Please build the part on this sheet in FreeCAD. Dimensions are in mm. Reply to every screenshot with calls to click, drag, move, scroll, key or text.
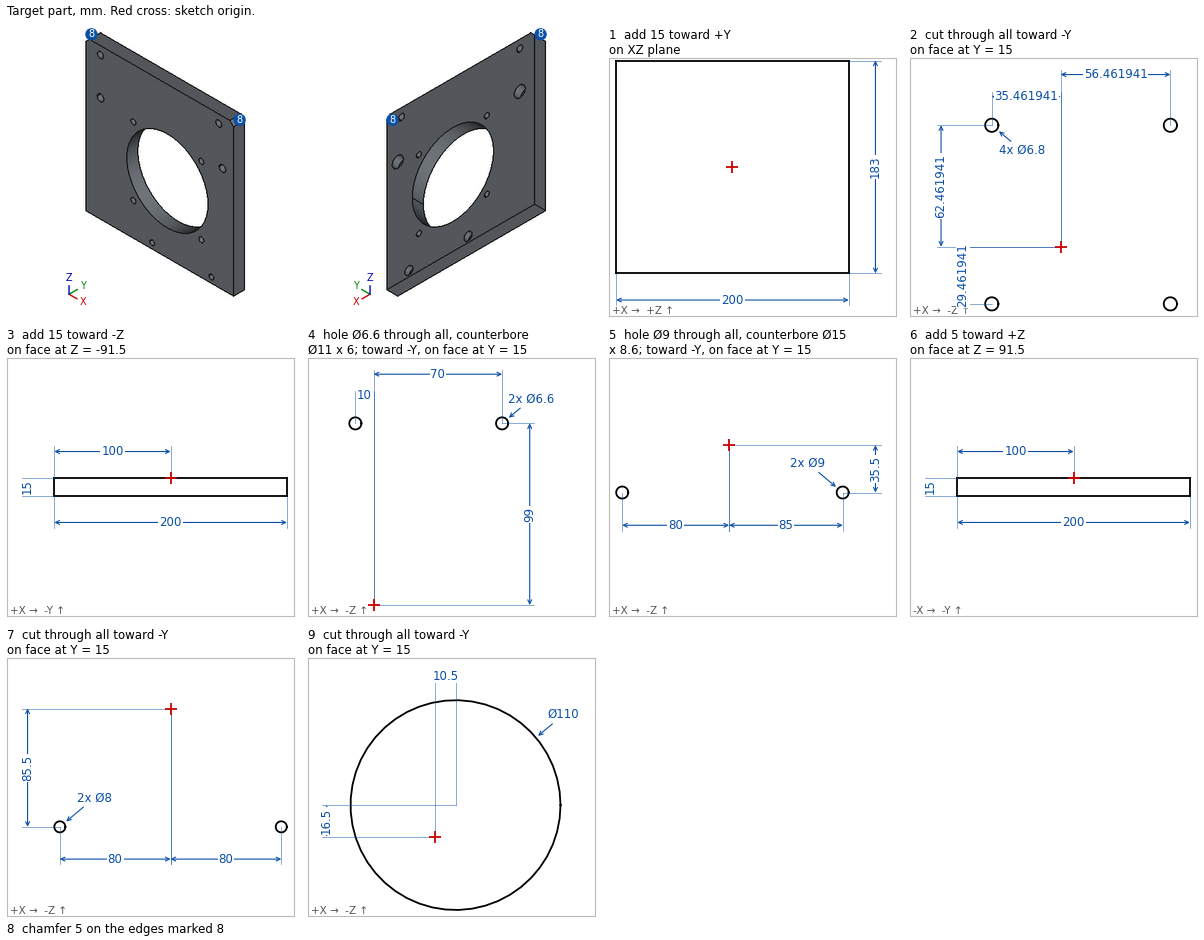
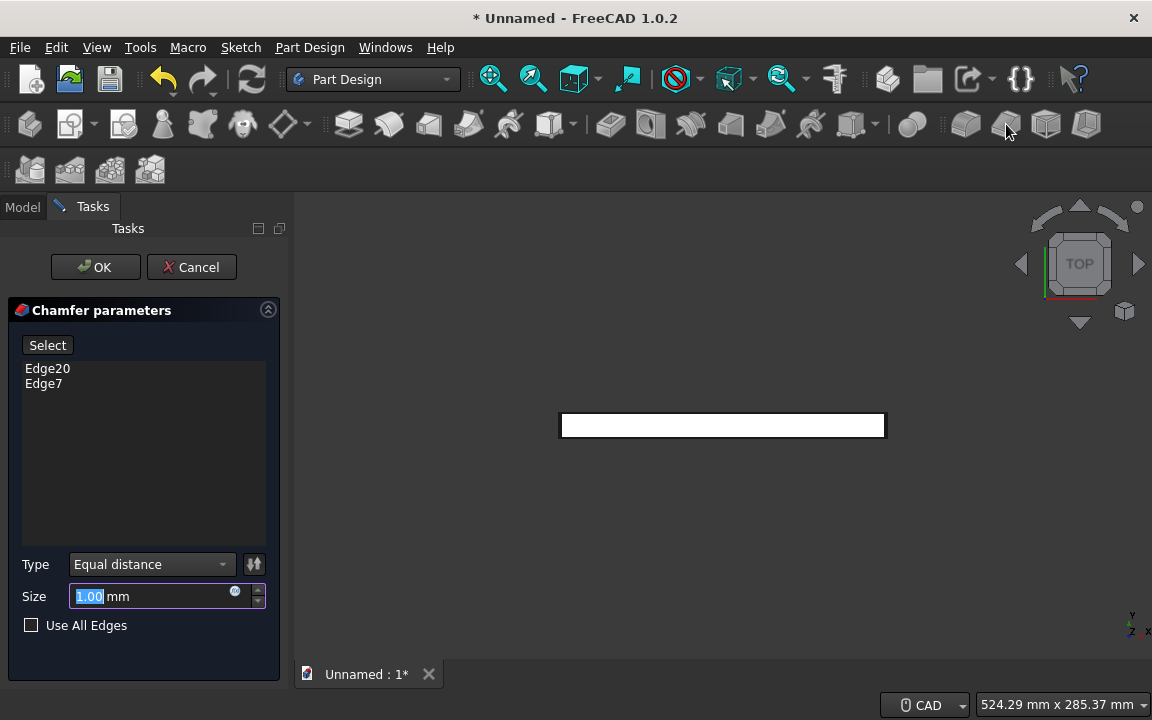
text(5)
key(Tab)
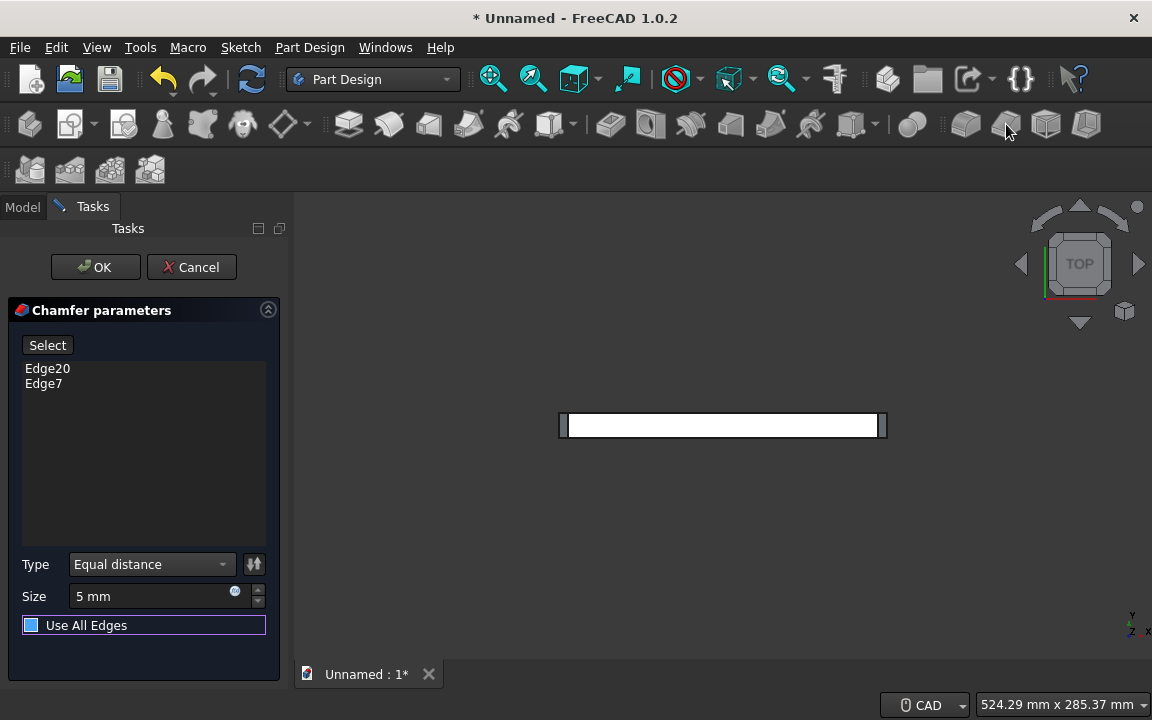
click(96, 267)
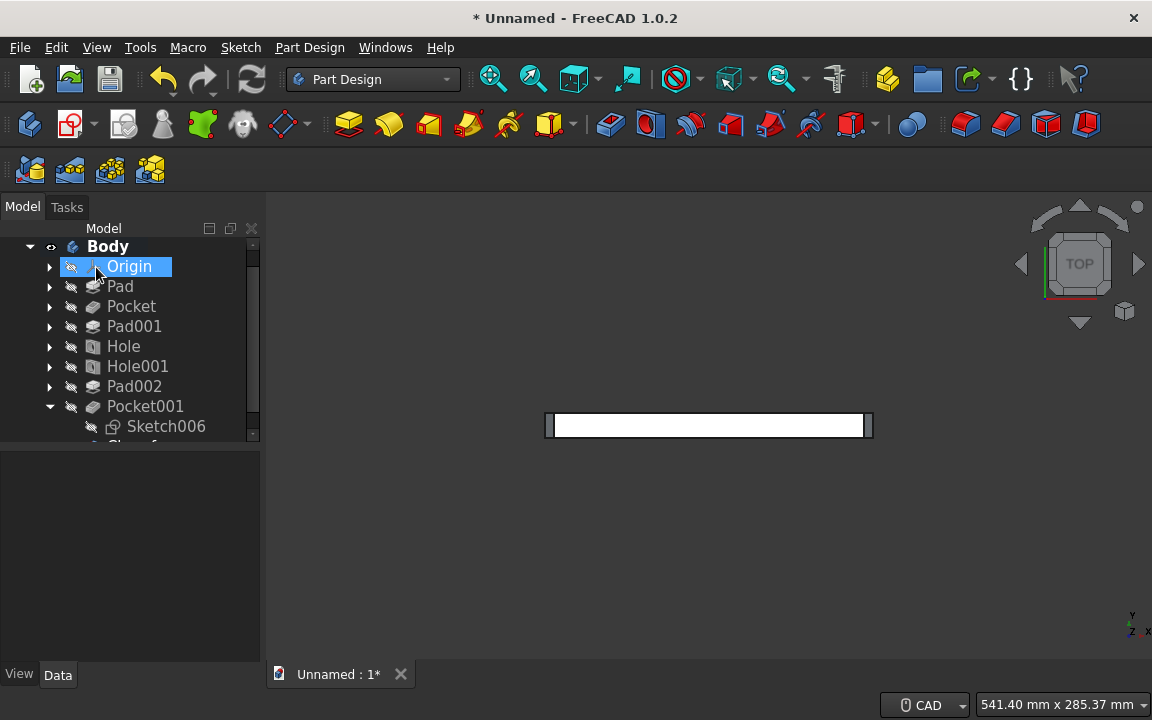
click(494, 80)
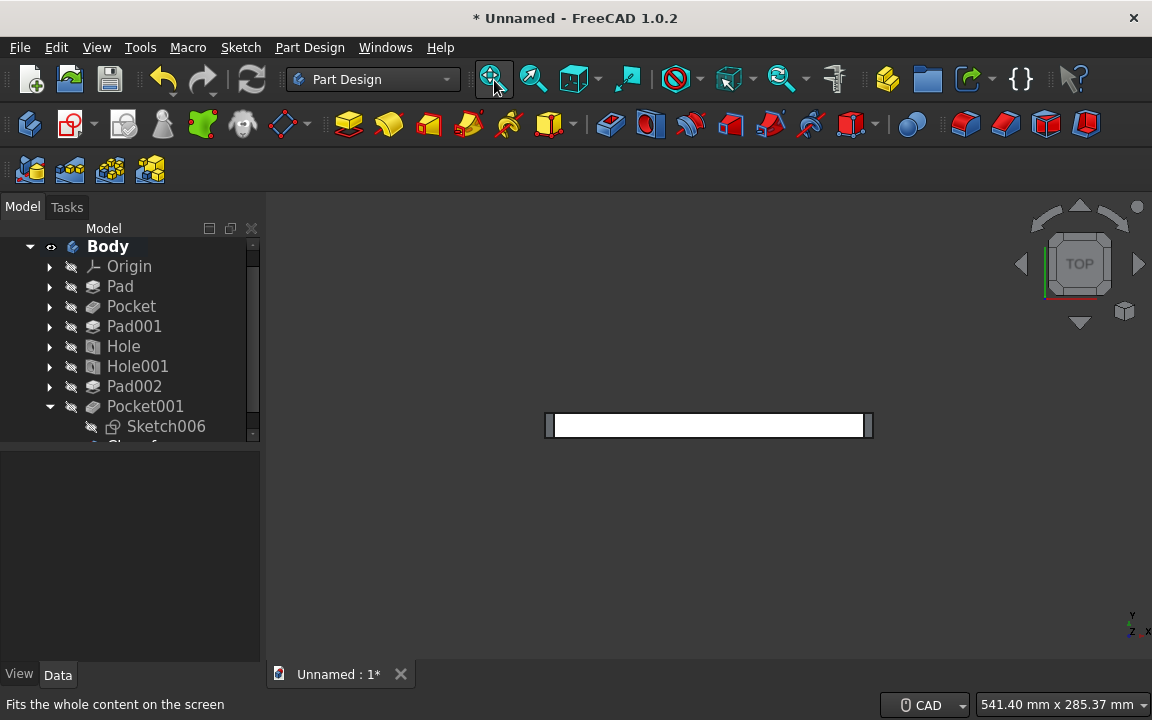
key(4)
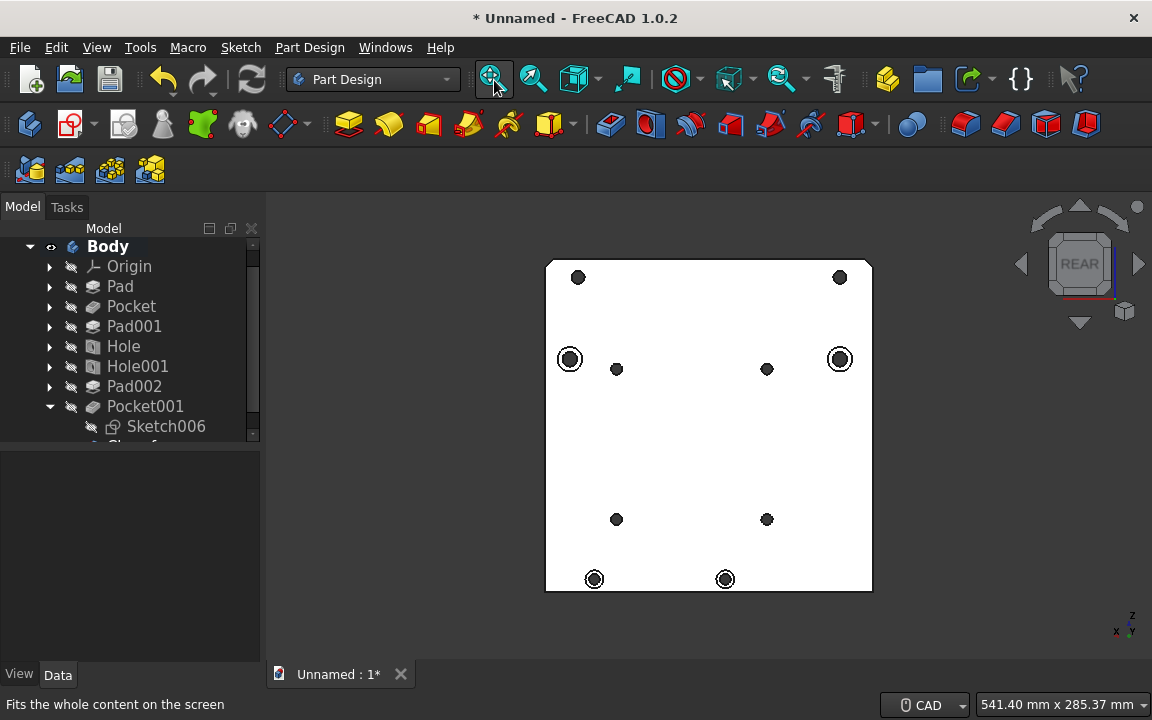
click(709, 425)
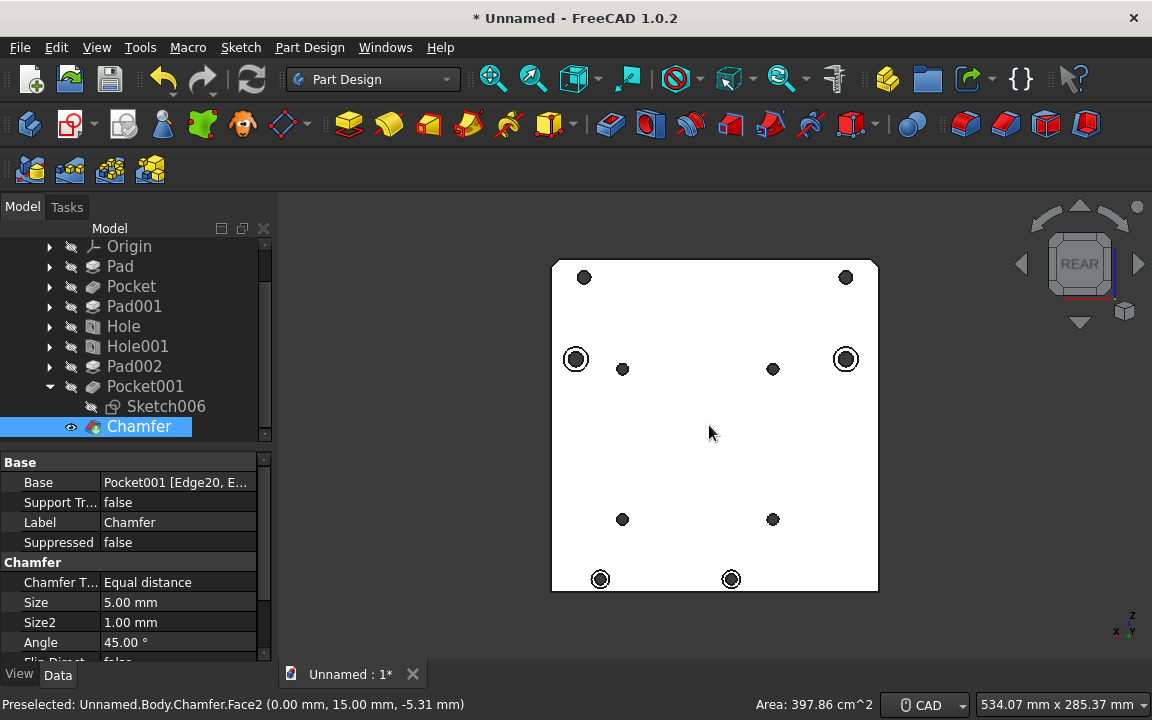
click(70, 124)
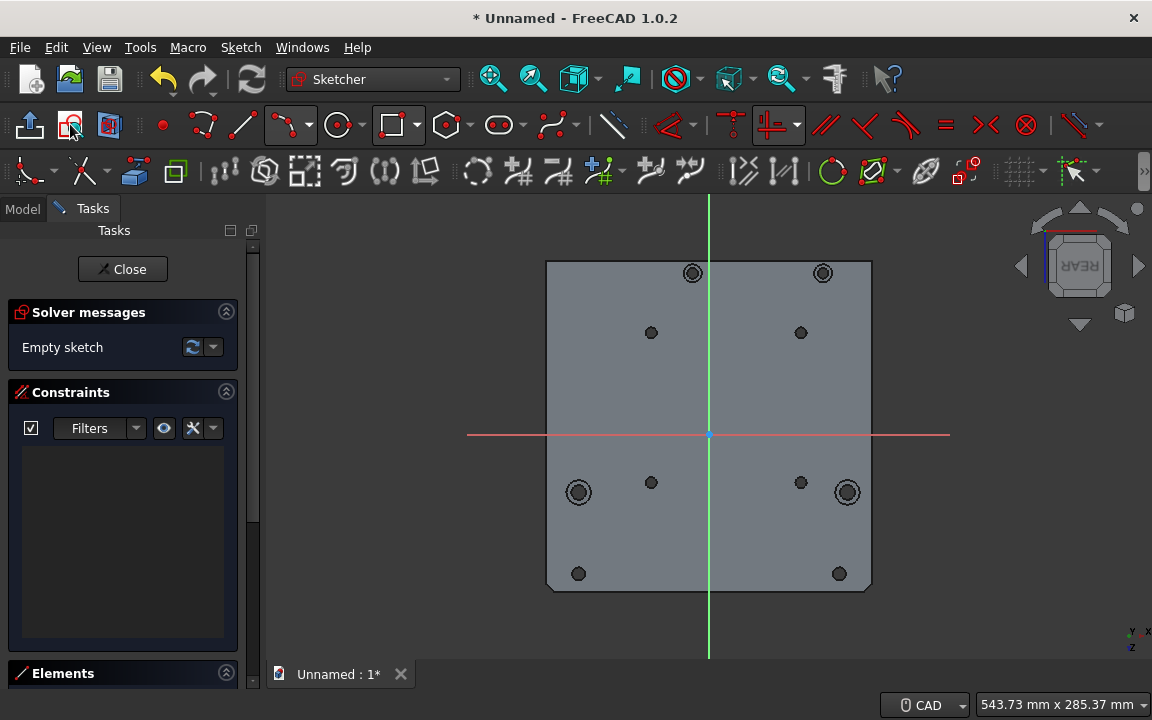
scroll(900, 370, up, 2)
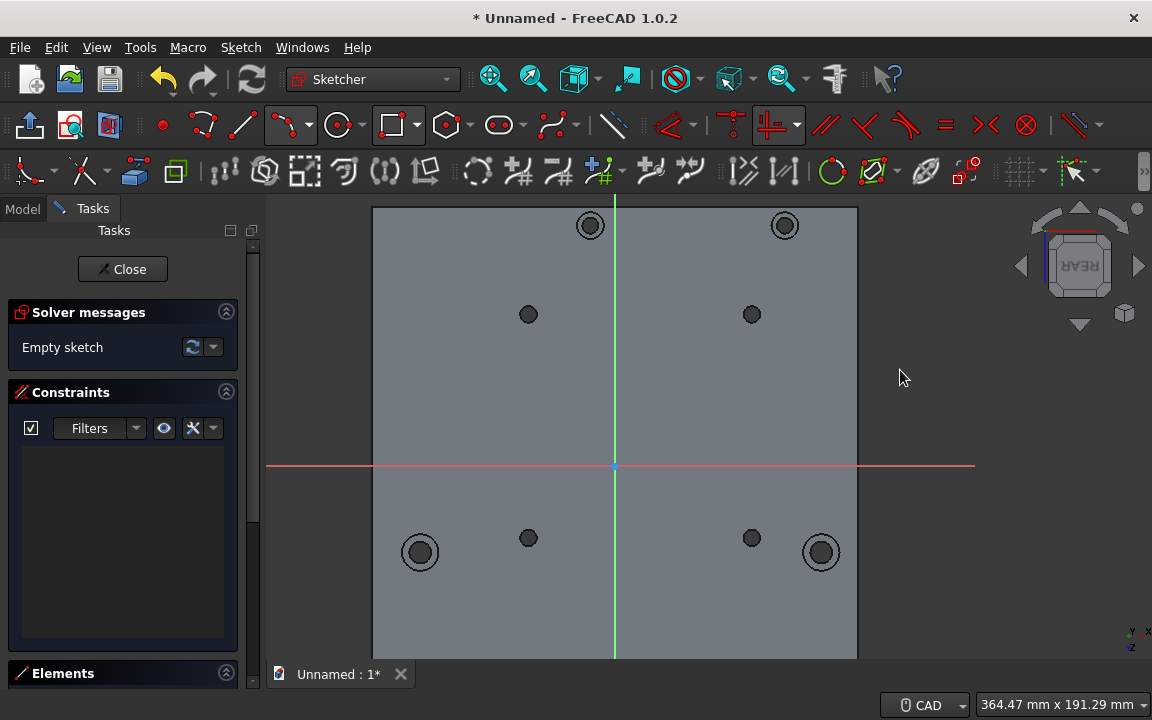
click(338, 126)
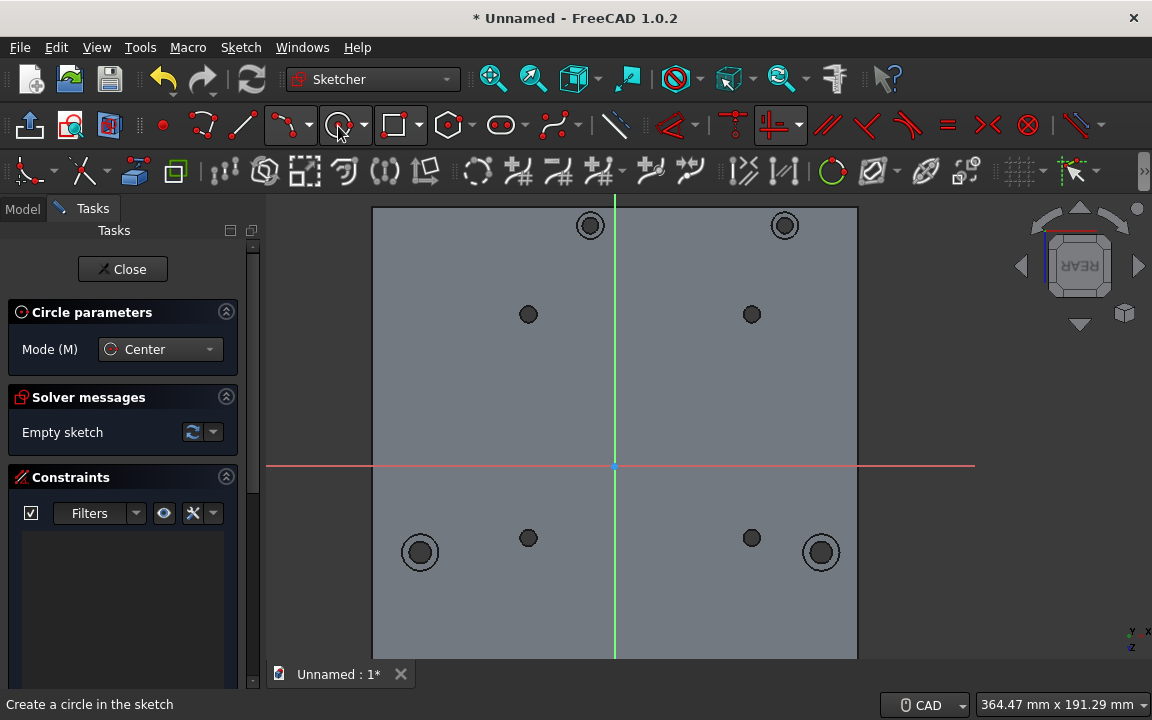
click(640, 426)
click(735, 332)
key(Escape)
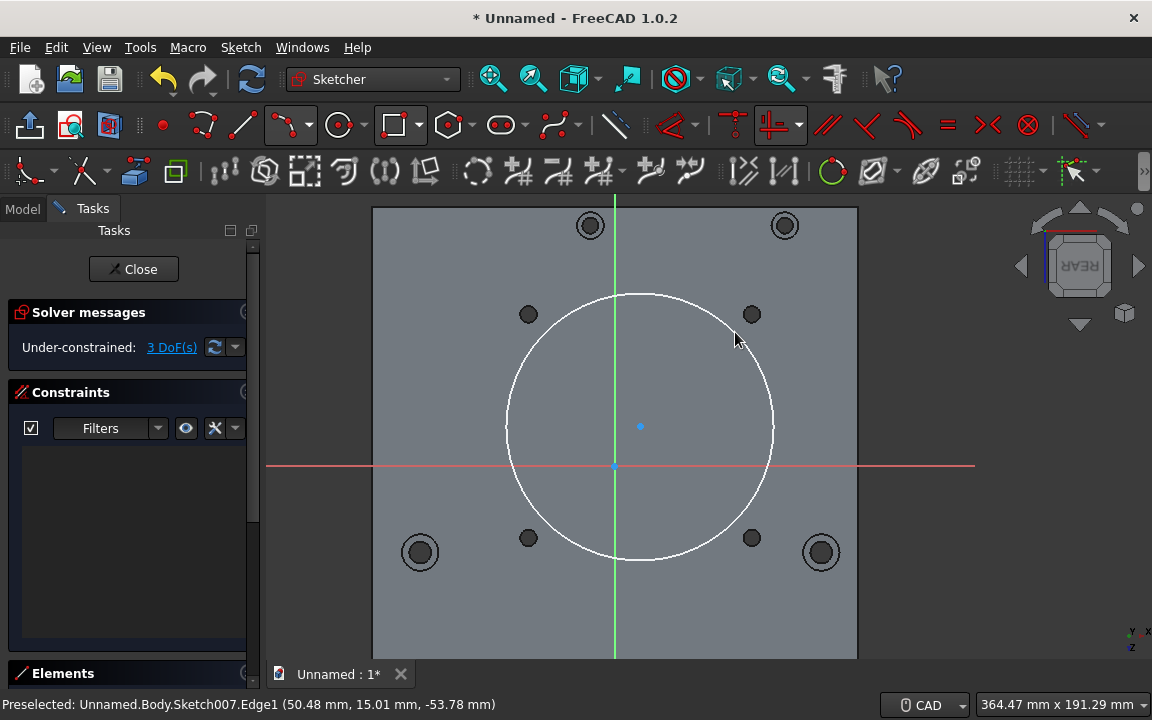
click(670, 126)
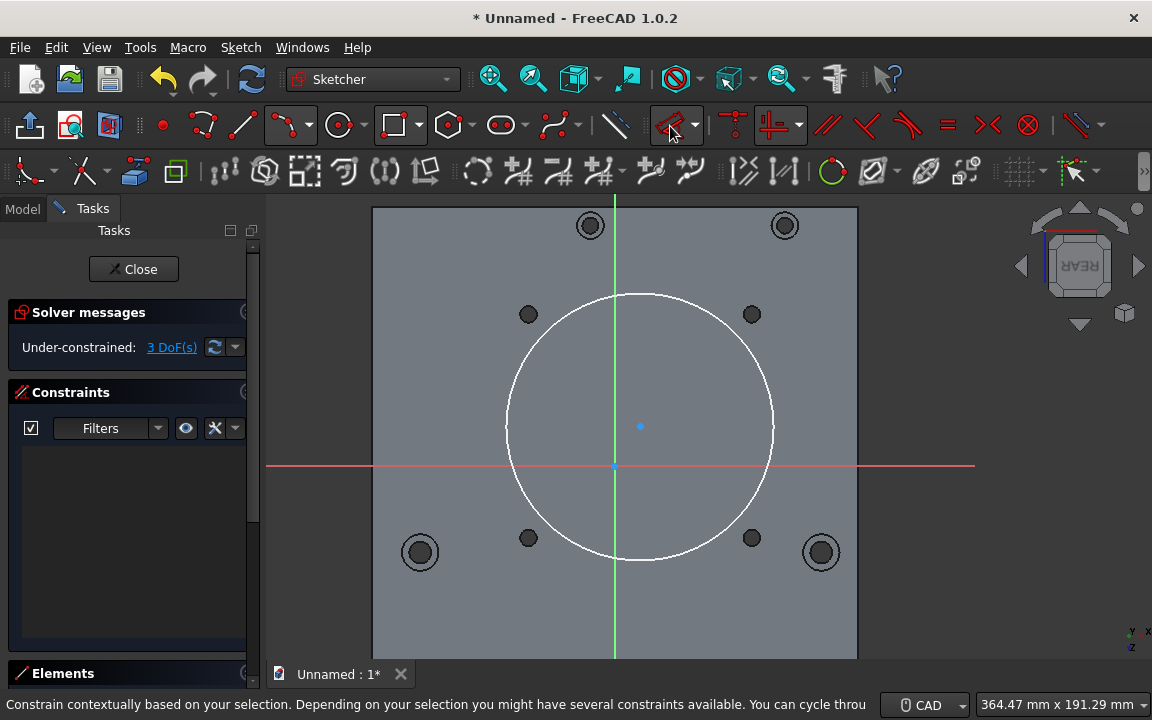
click(734, 332)
click(757, 309)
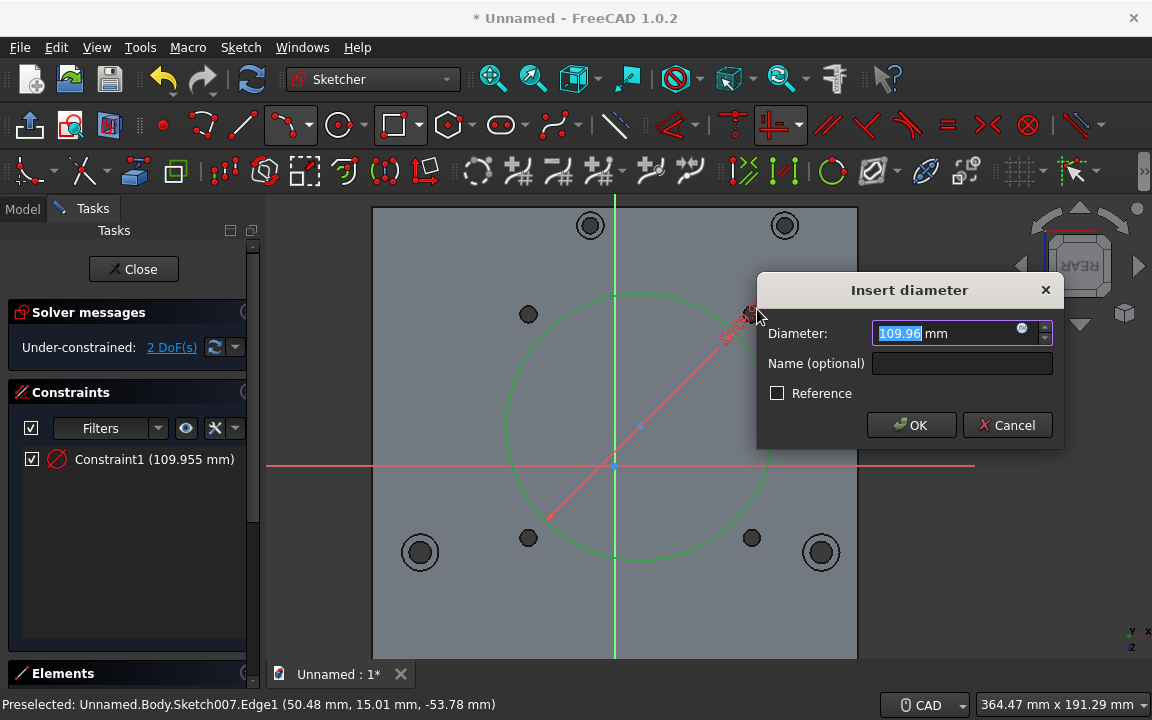
text(110)
key(Return)